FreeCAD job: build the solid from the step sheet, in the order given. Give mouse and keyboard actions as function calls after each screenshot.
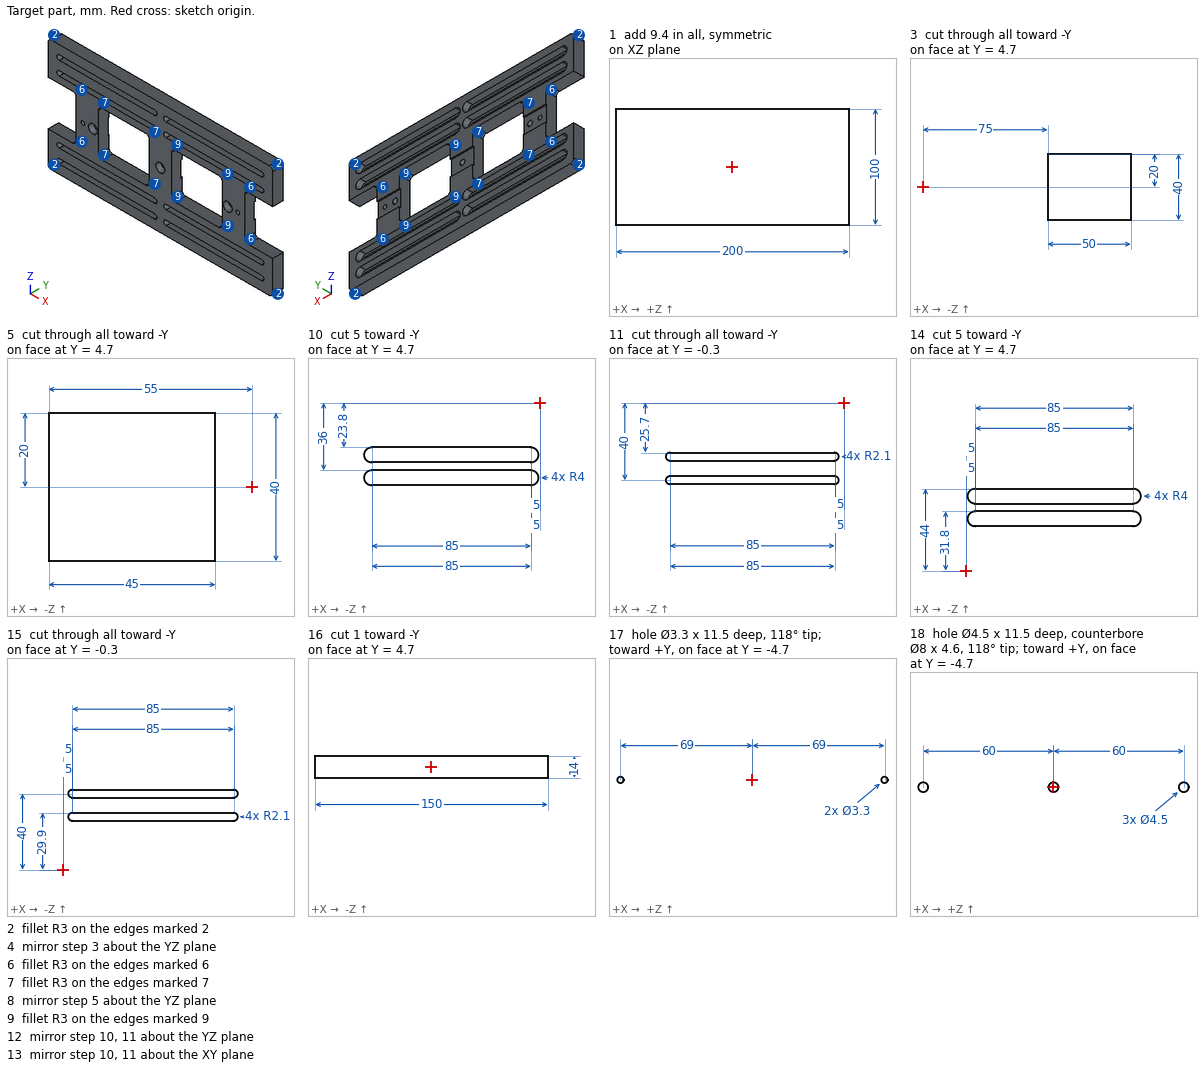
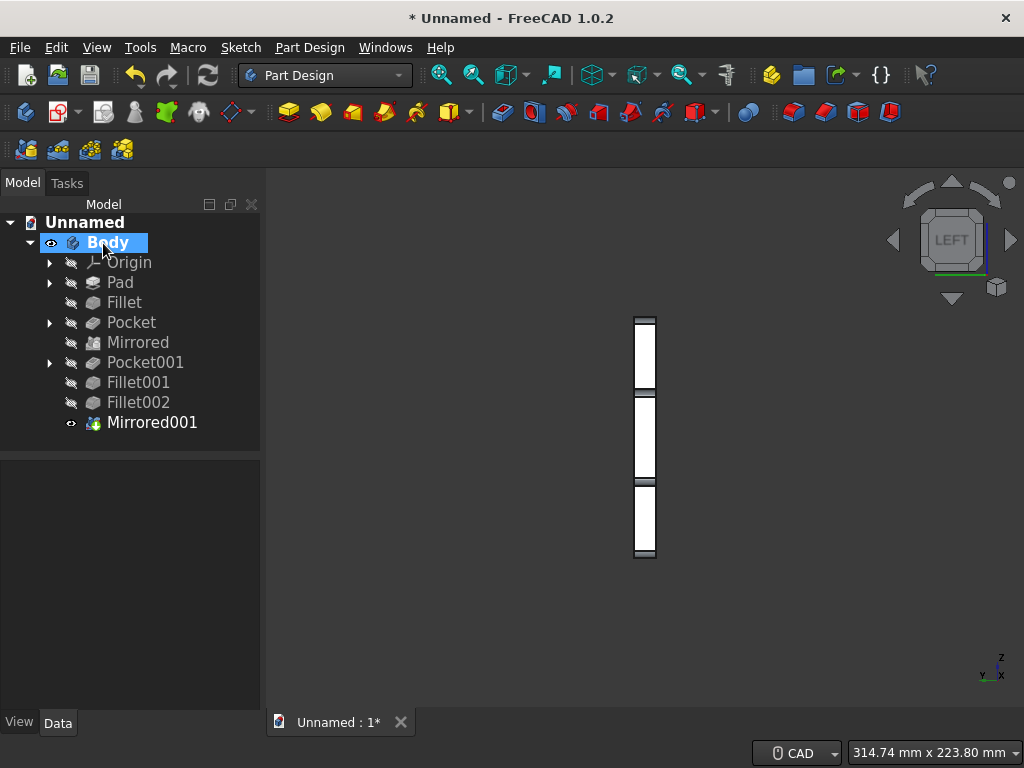
key(0)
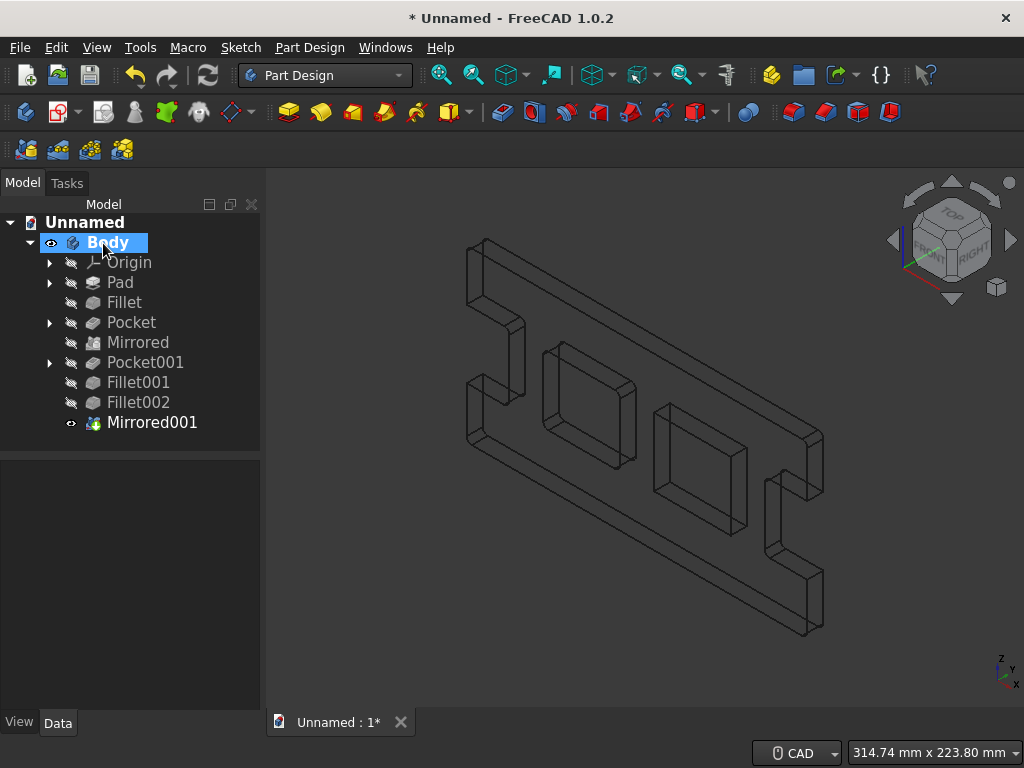
click(739, 451)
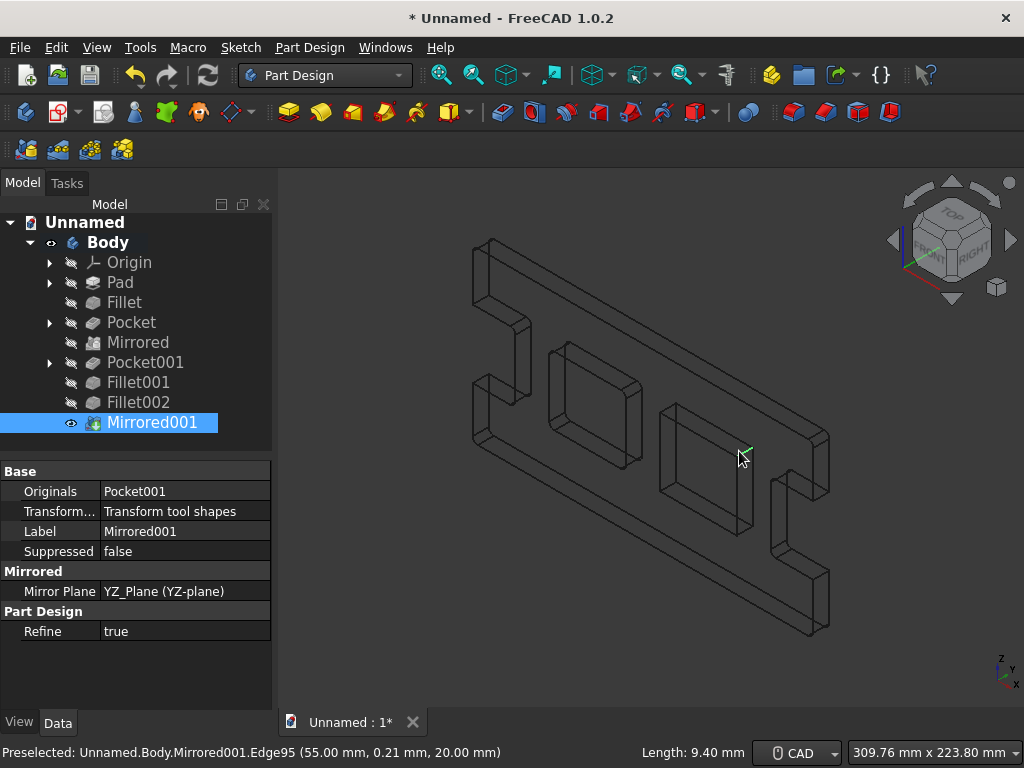
click(745, 530, ctrl)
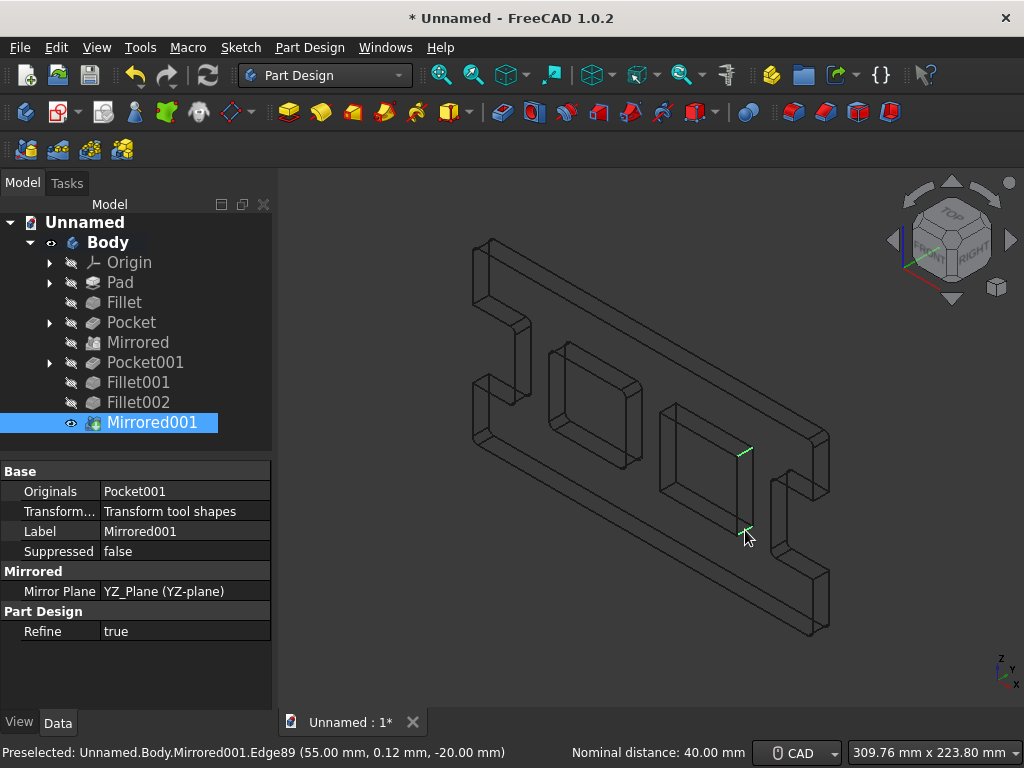
click(668, 486, ctrl)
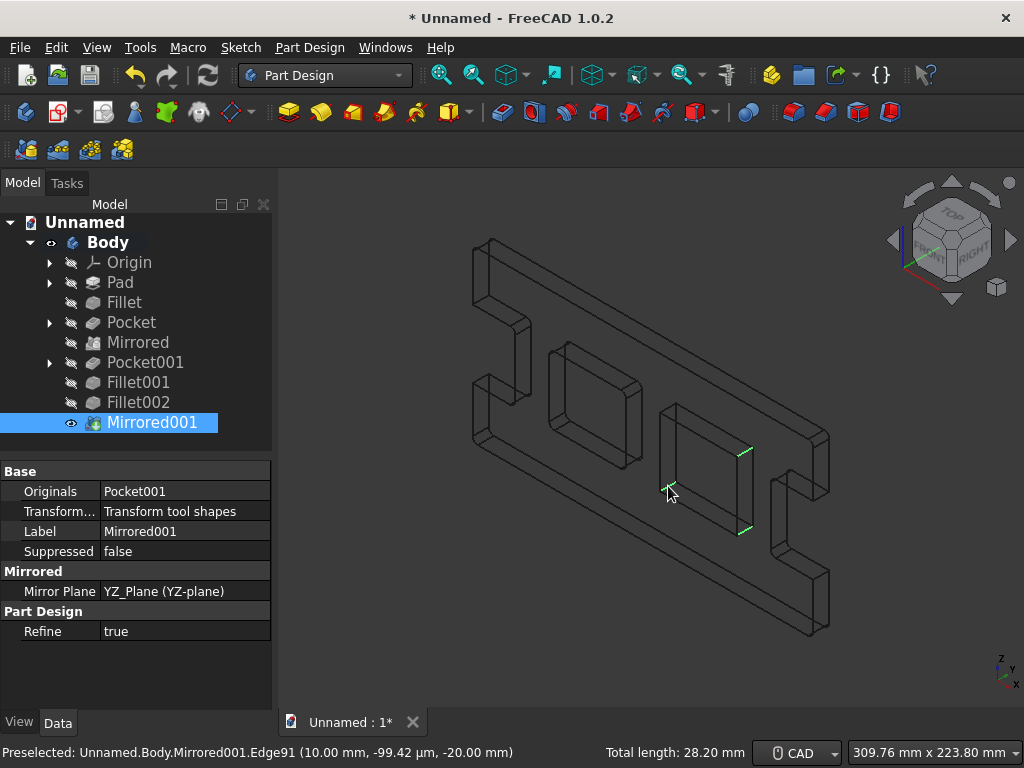
click(668, 407, ctrl)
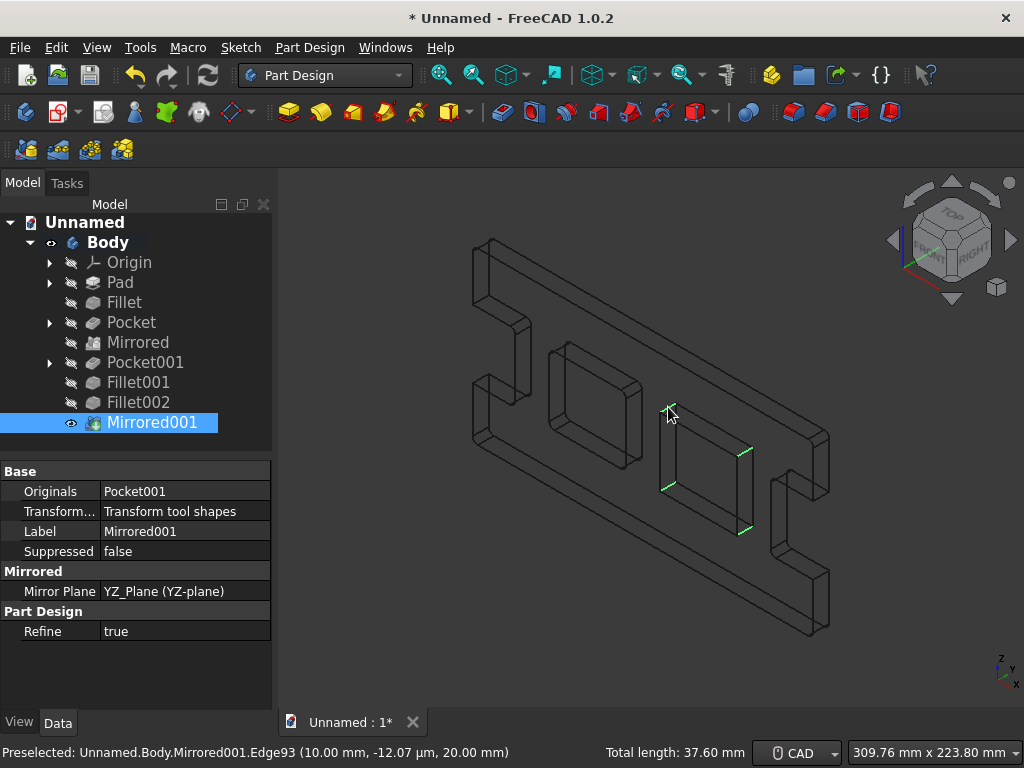
key(v)
key(1)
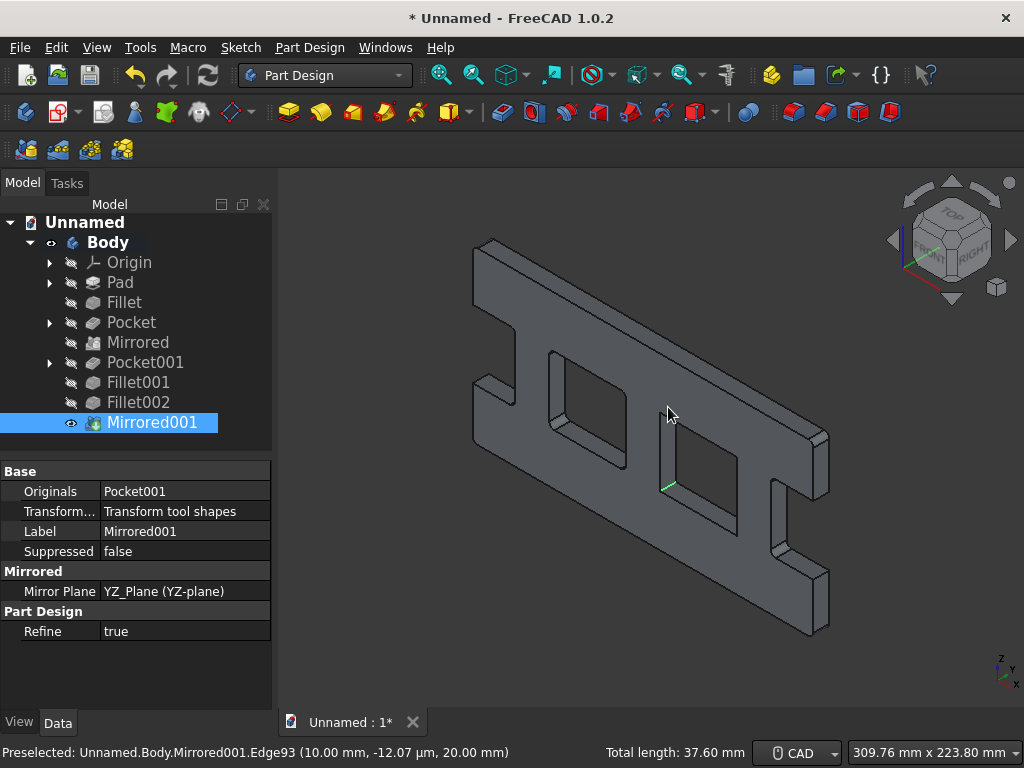
click(794, 112)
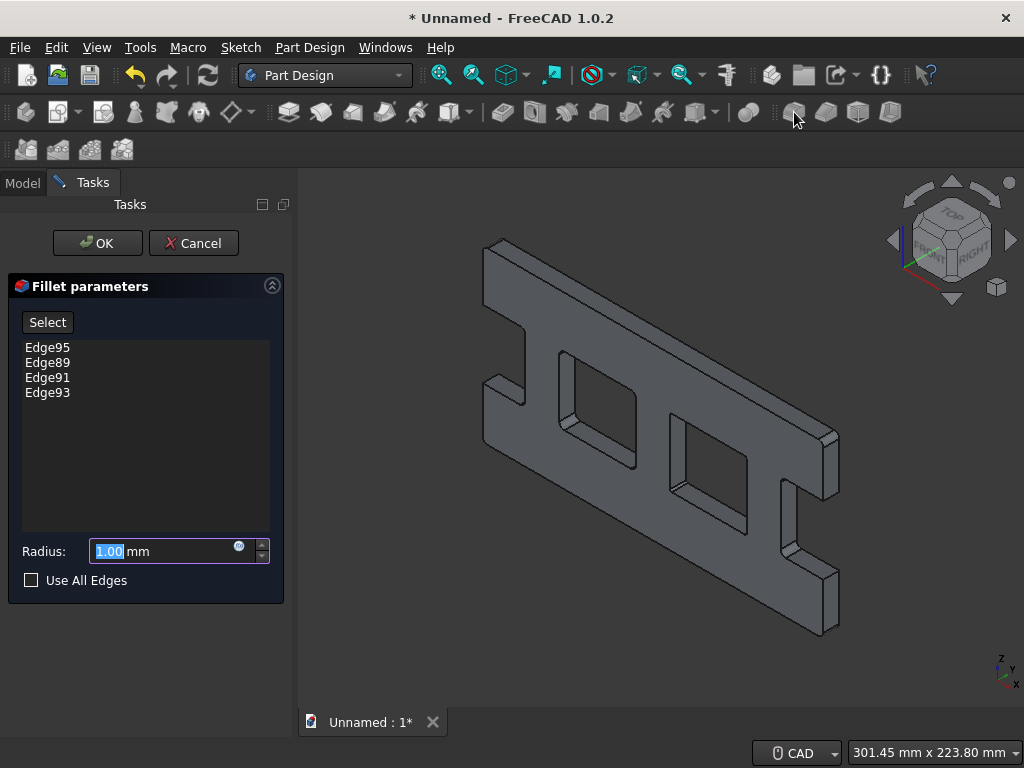
text(3)
key(Tab)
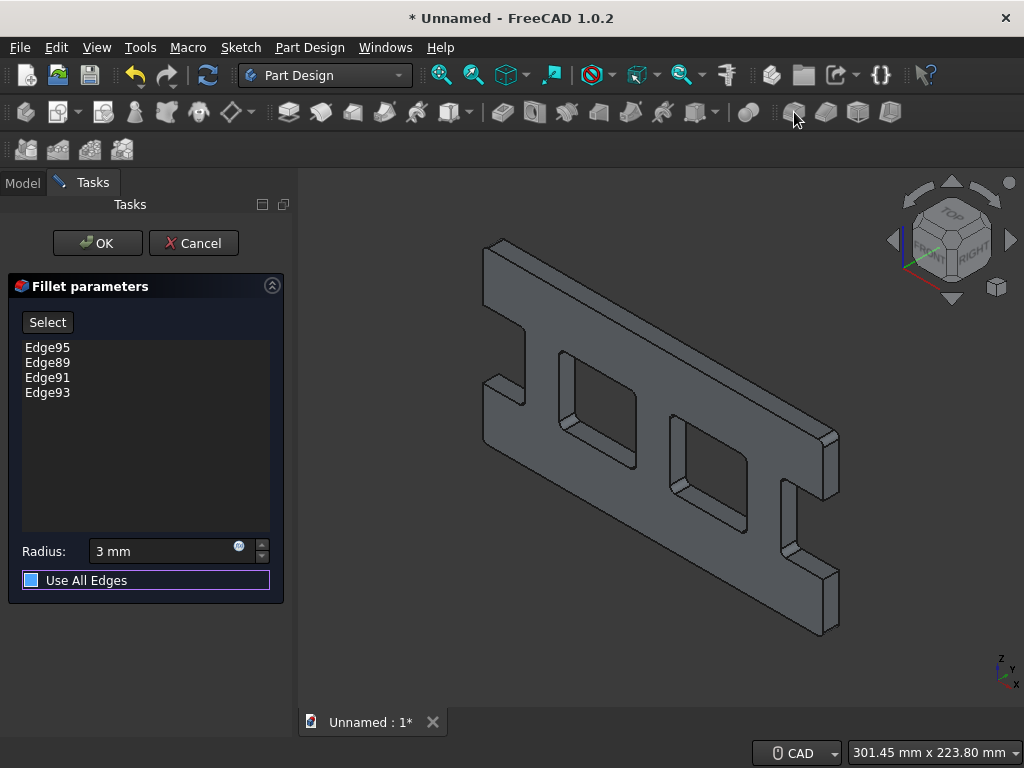
click(98, 243)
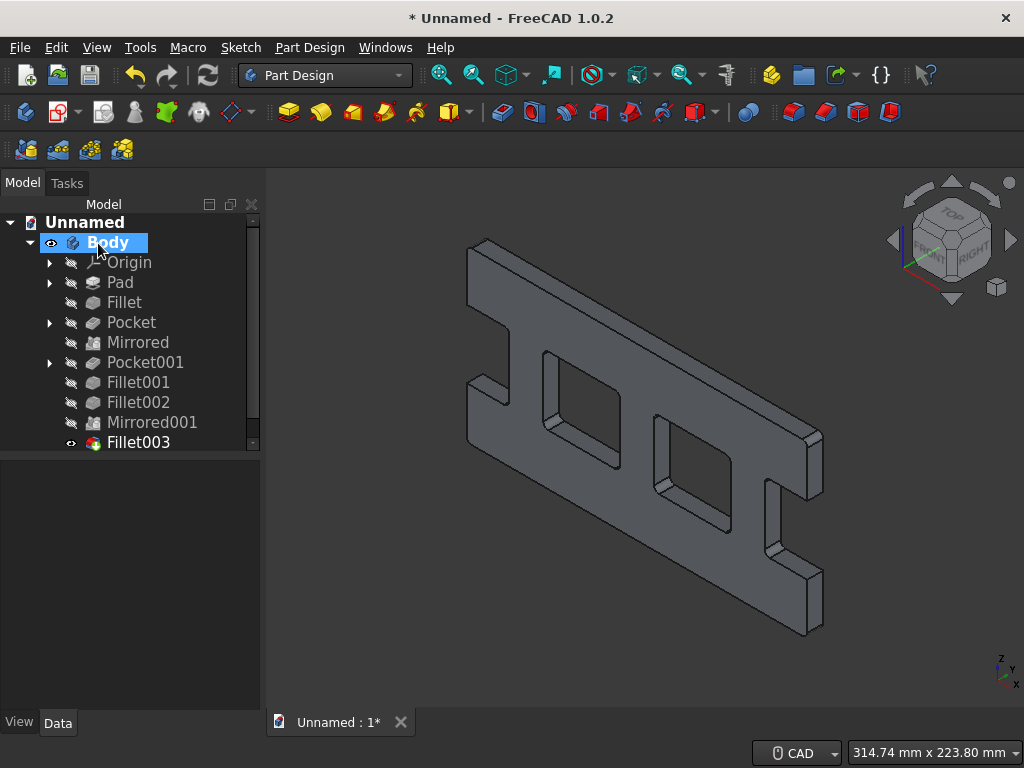
key(4)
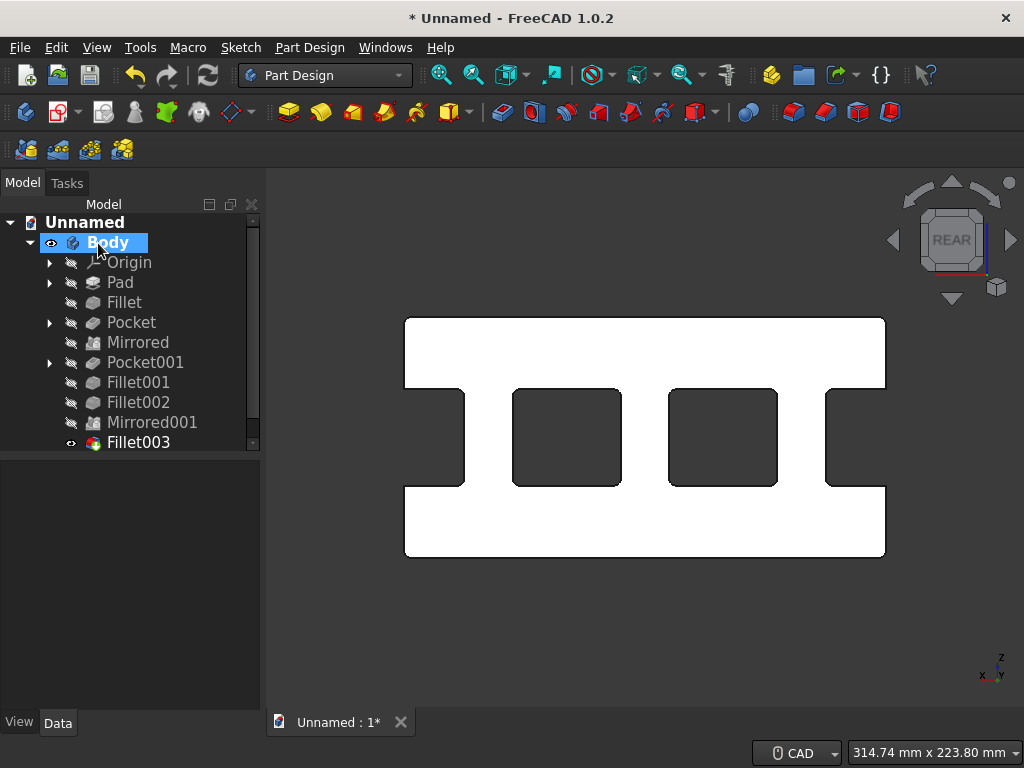
click(645, 505)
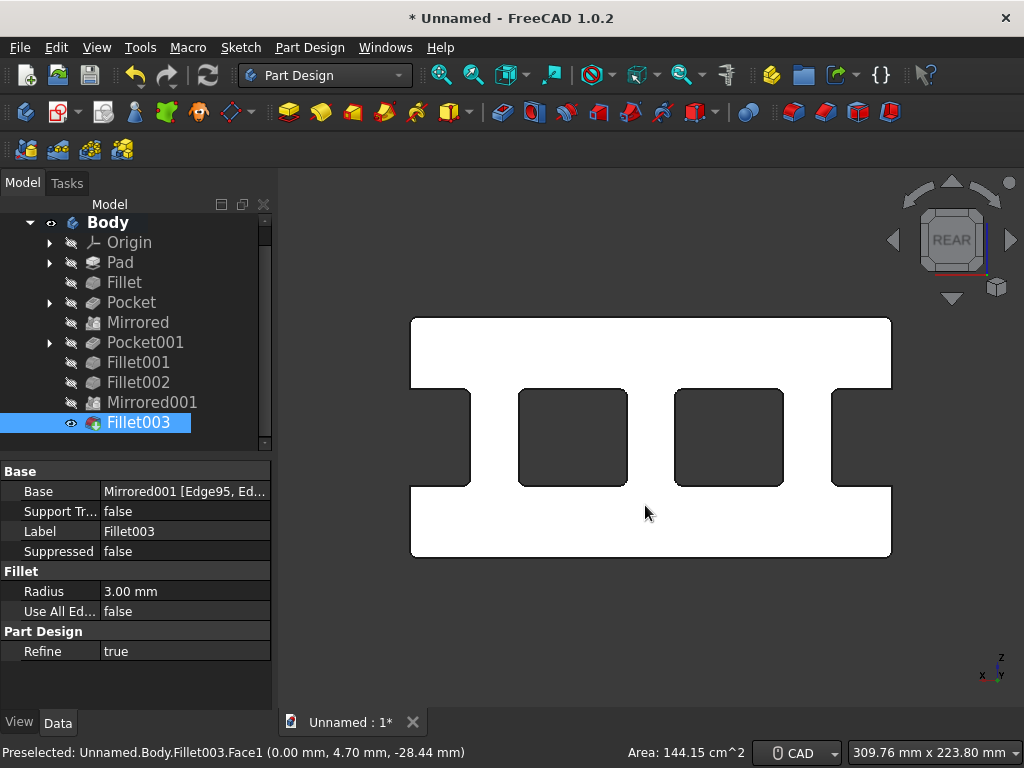
click(58, 112)